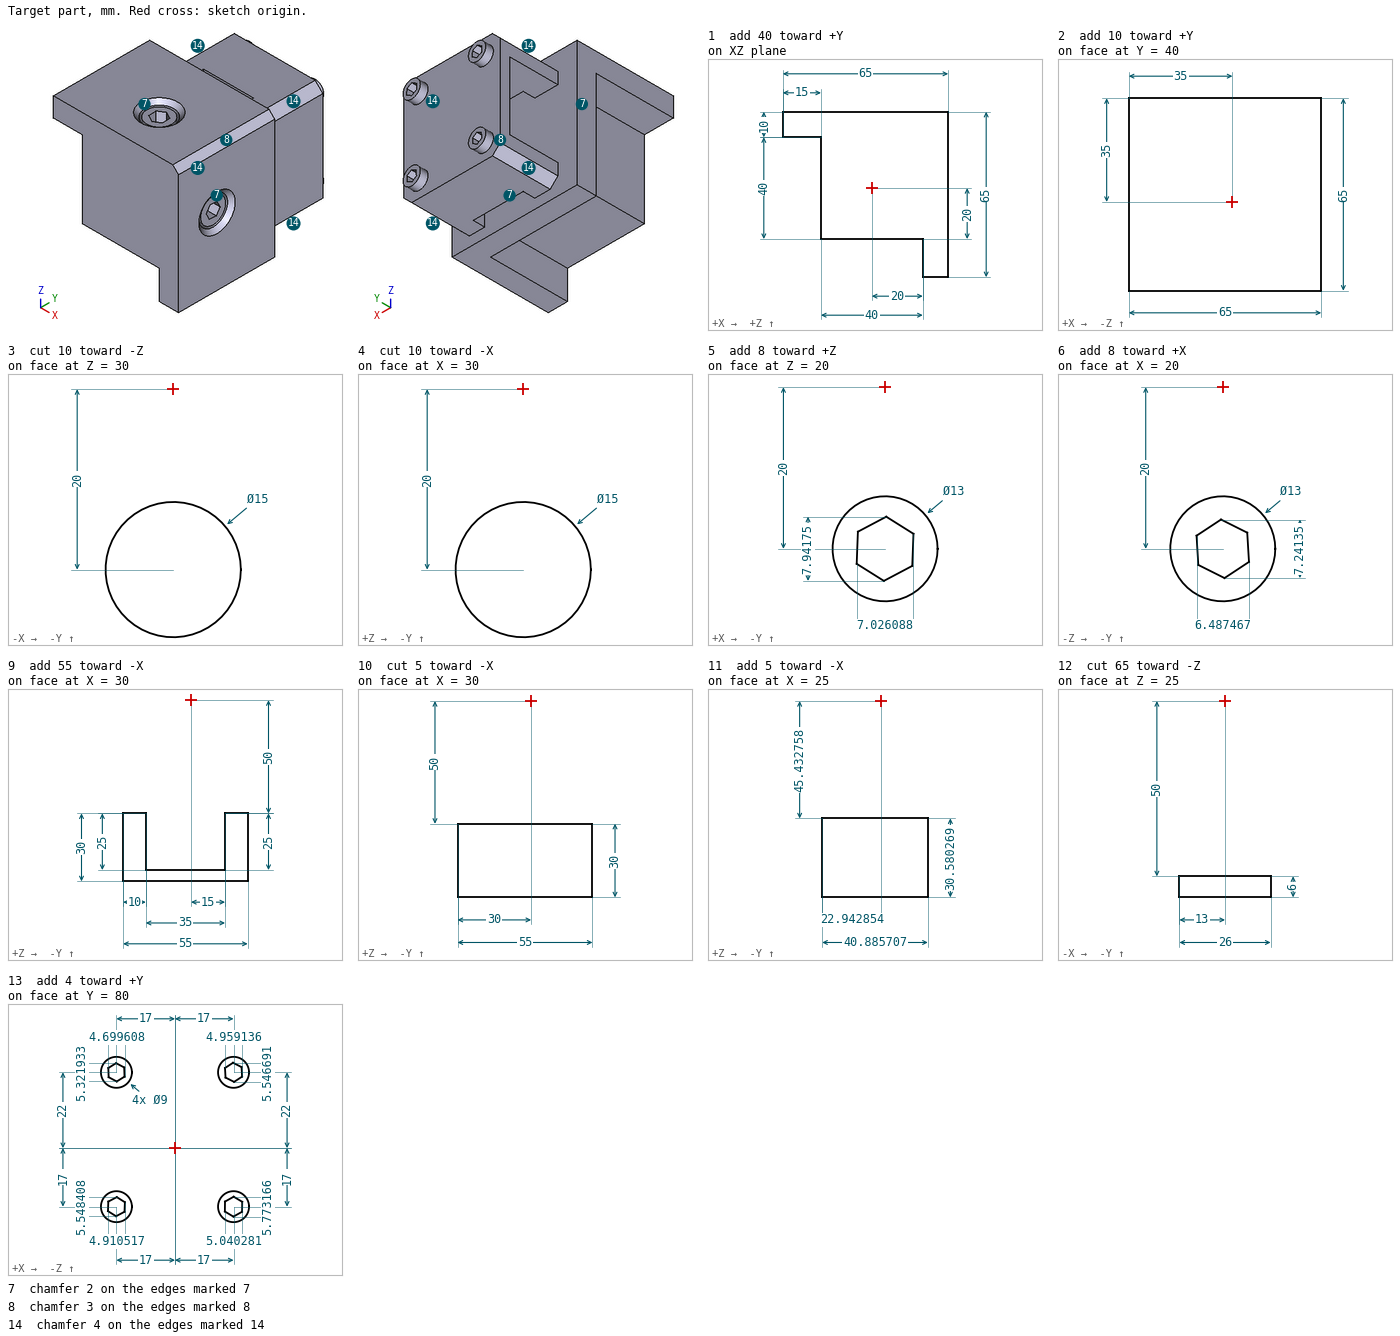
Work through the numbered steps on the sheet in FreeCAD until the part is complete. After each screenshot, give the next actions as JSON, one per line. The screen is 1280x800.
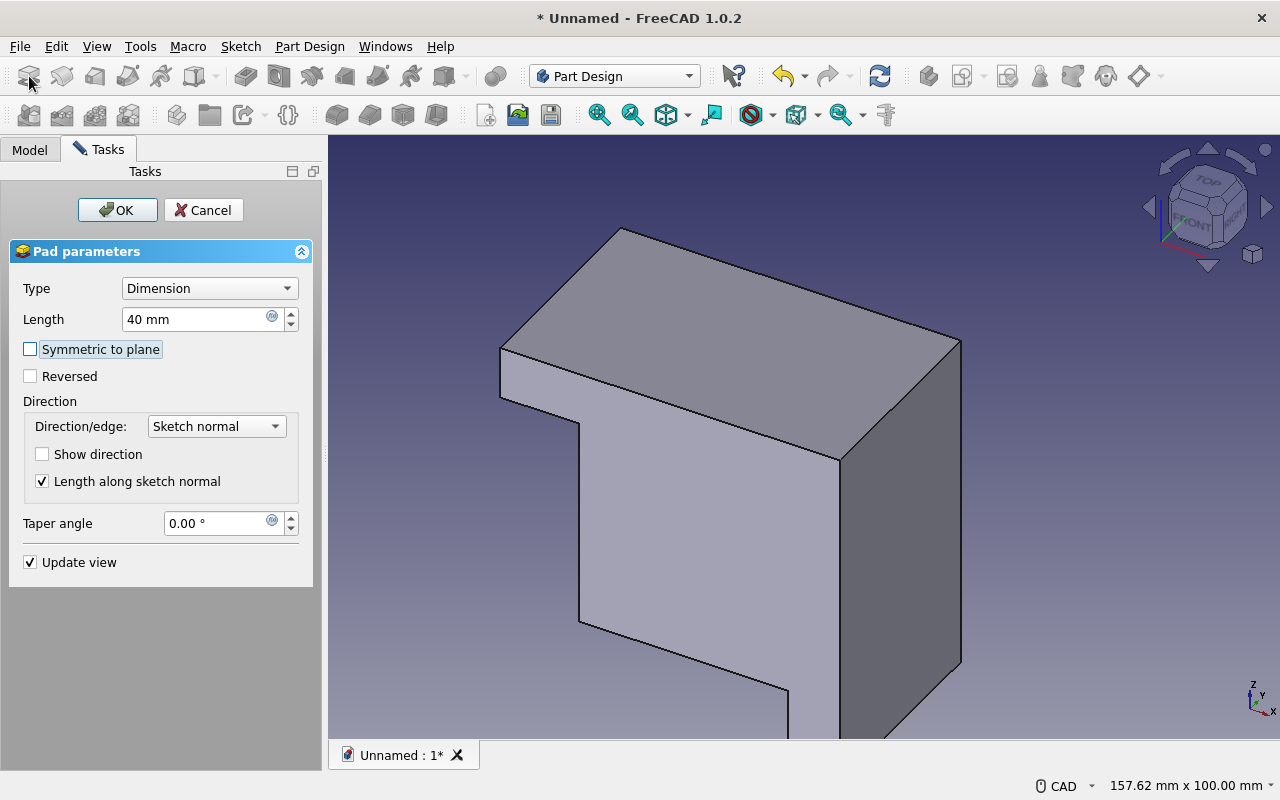
{"action": "left_click", "coordinate": [31, 376]}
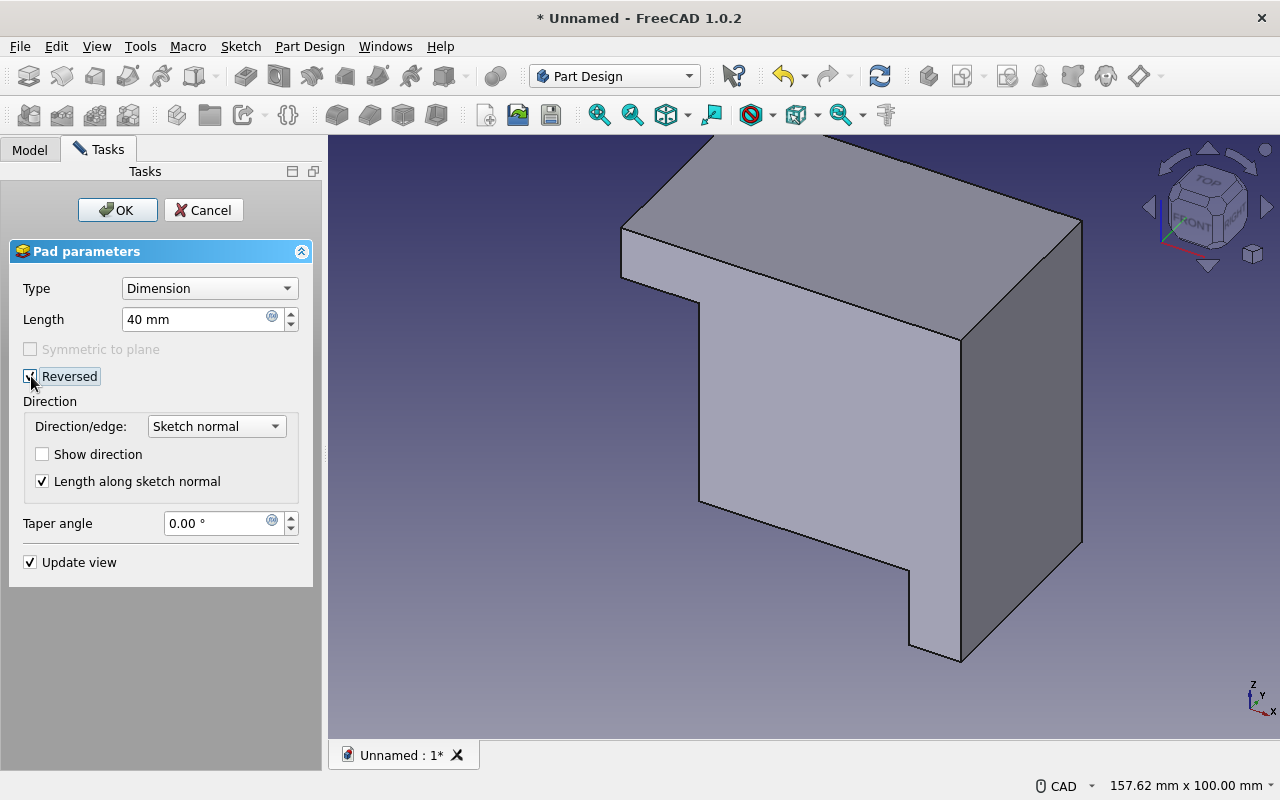
{"action": "left_click", "coordinate": [118, 210]}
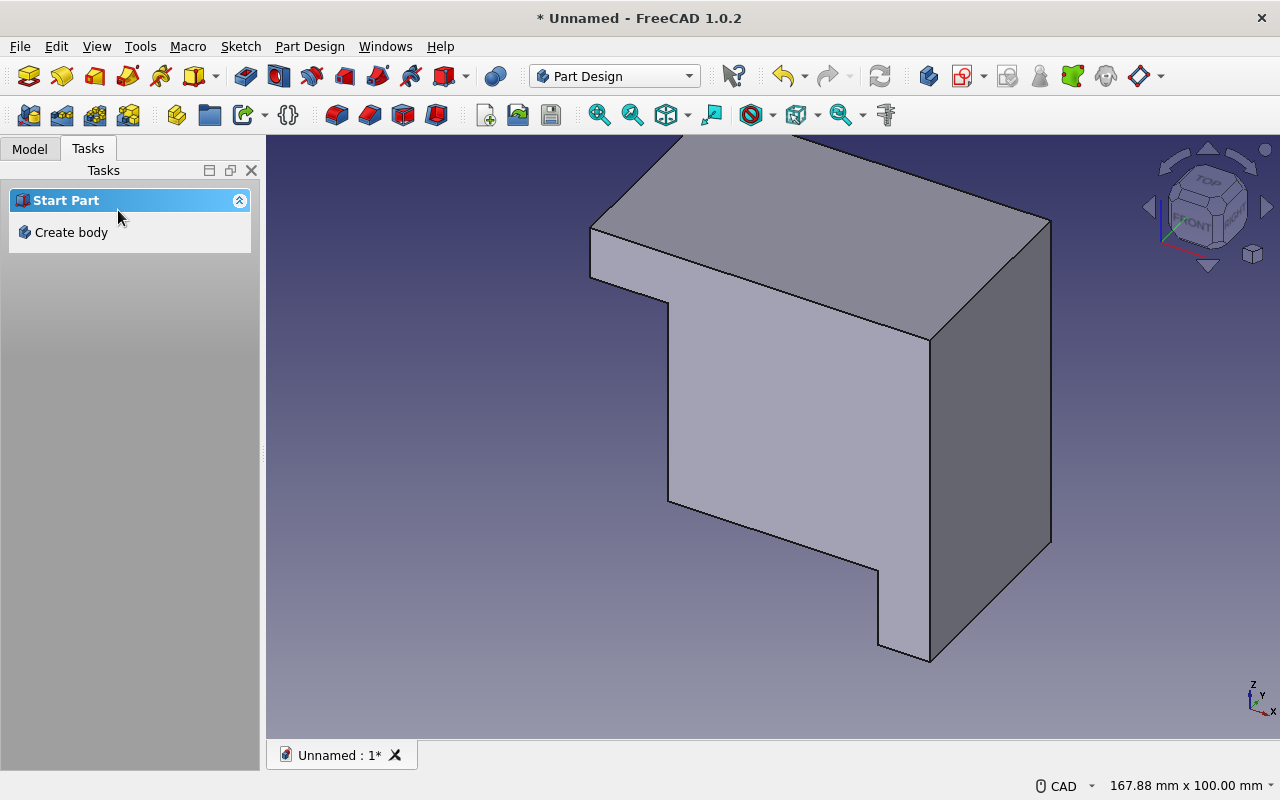
{"action": "left_click", "coordinate": [600, 116]}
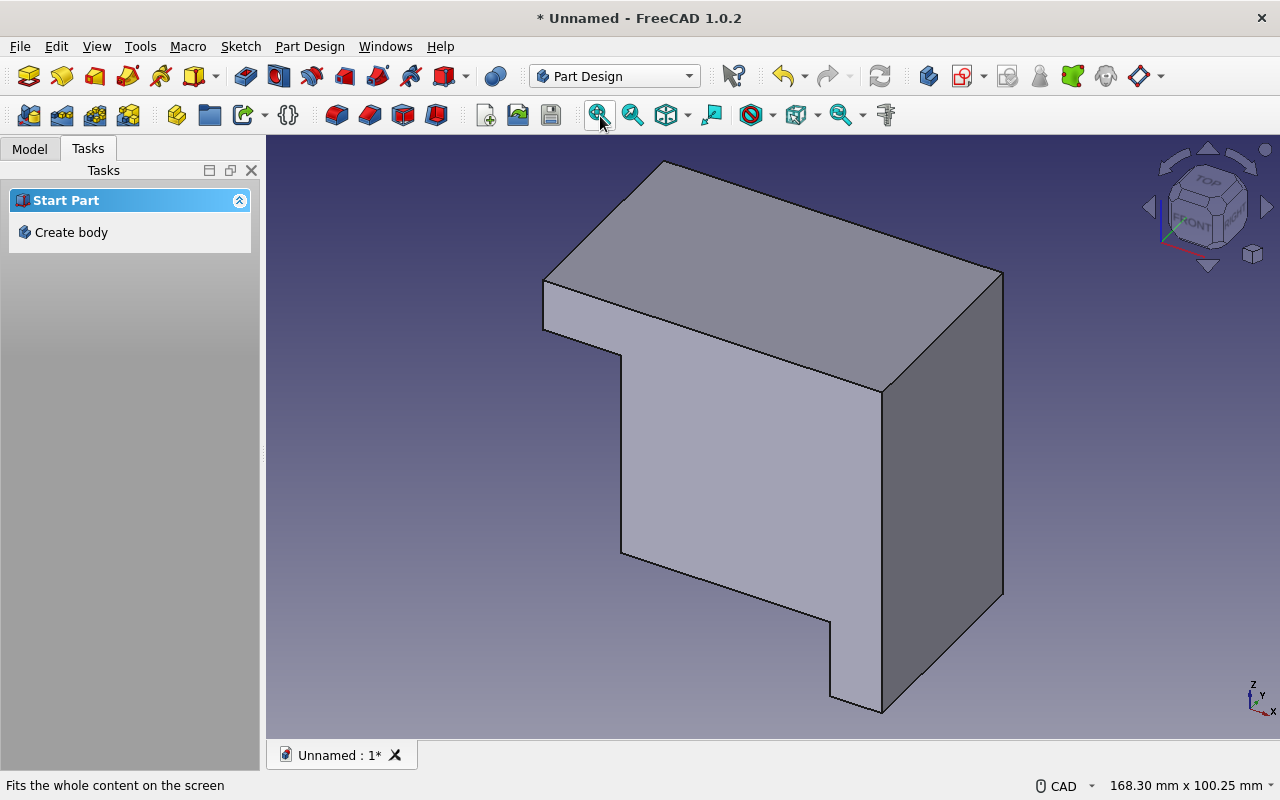
{"action": "key", "text": "4"}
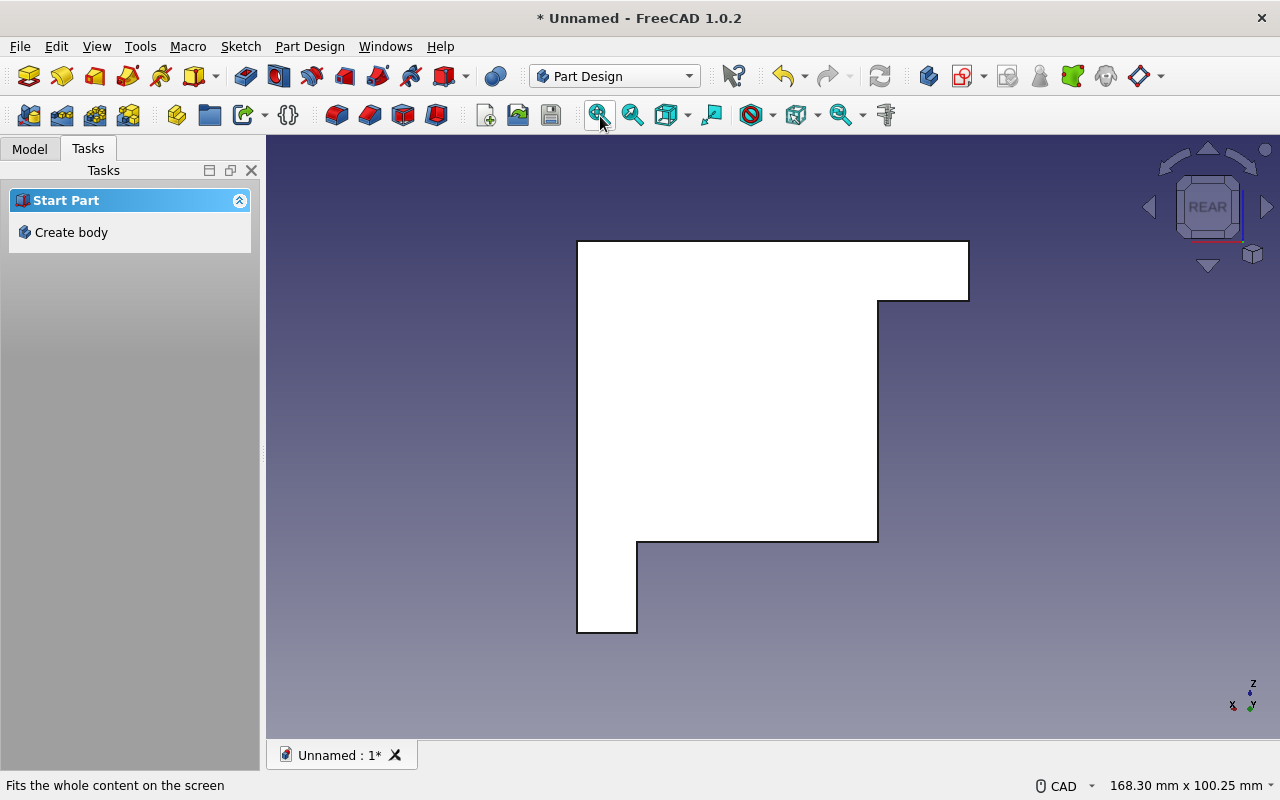
{"action": "left_click", "coordinate": [717, 380]}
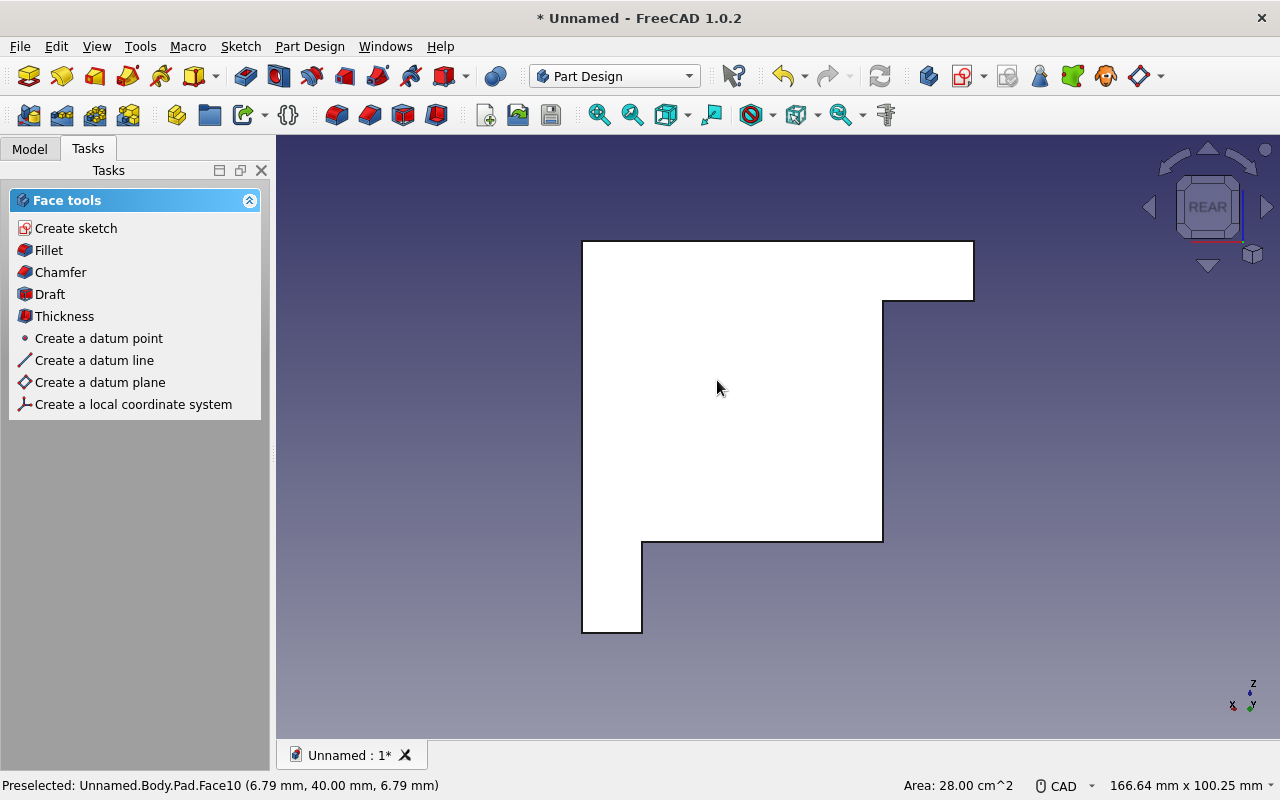
{"action": "left_click", "coordinate": [962, 76]}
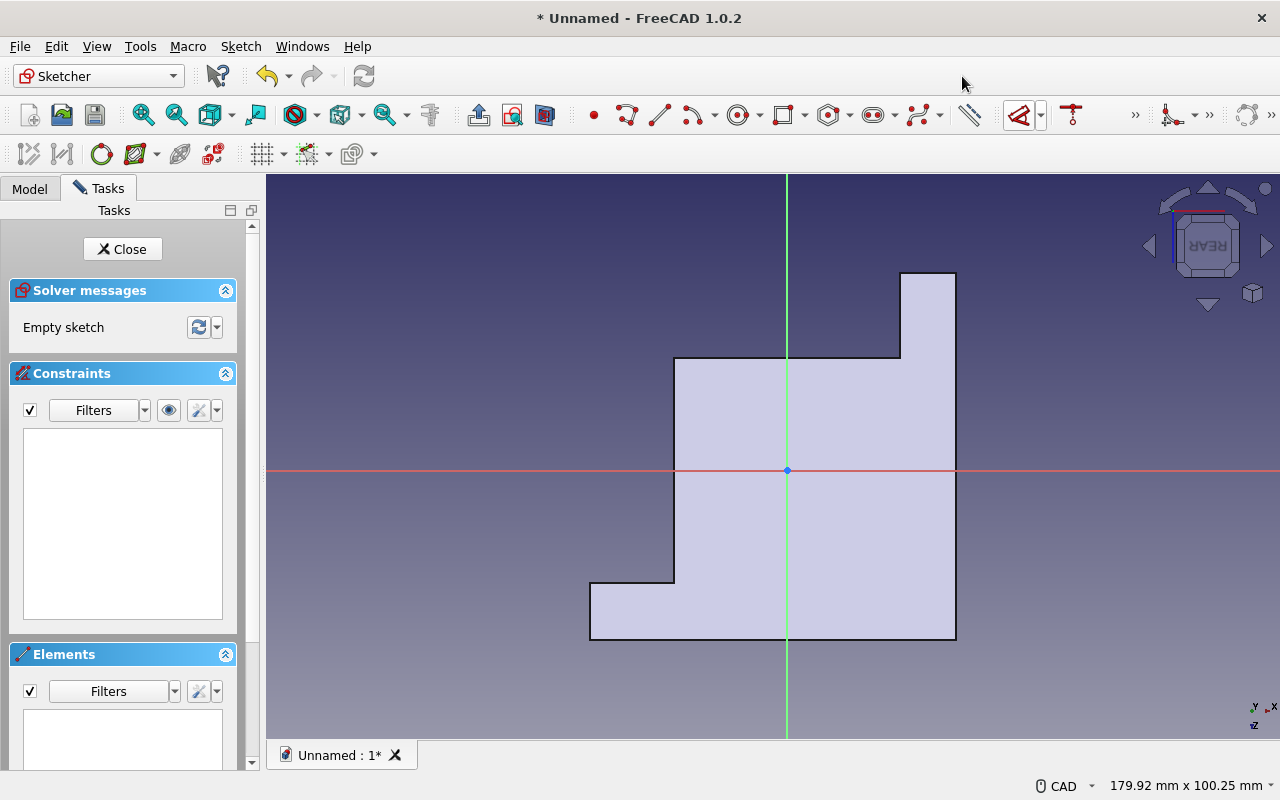
{"action": "left_click", "coordinate": [782, 116]}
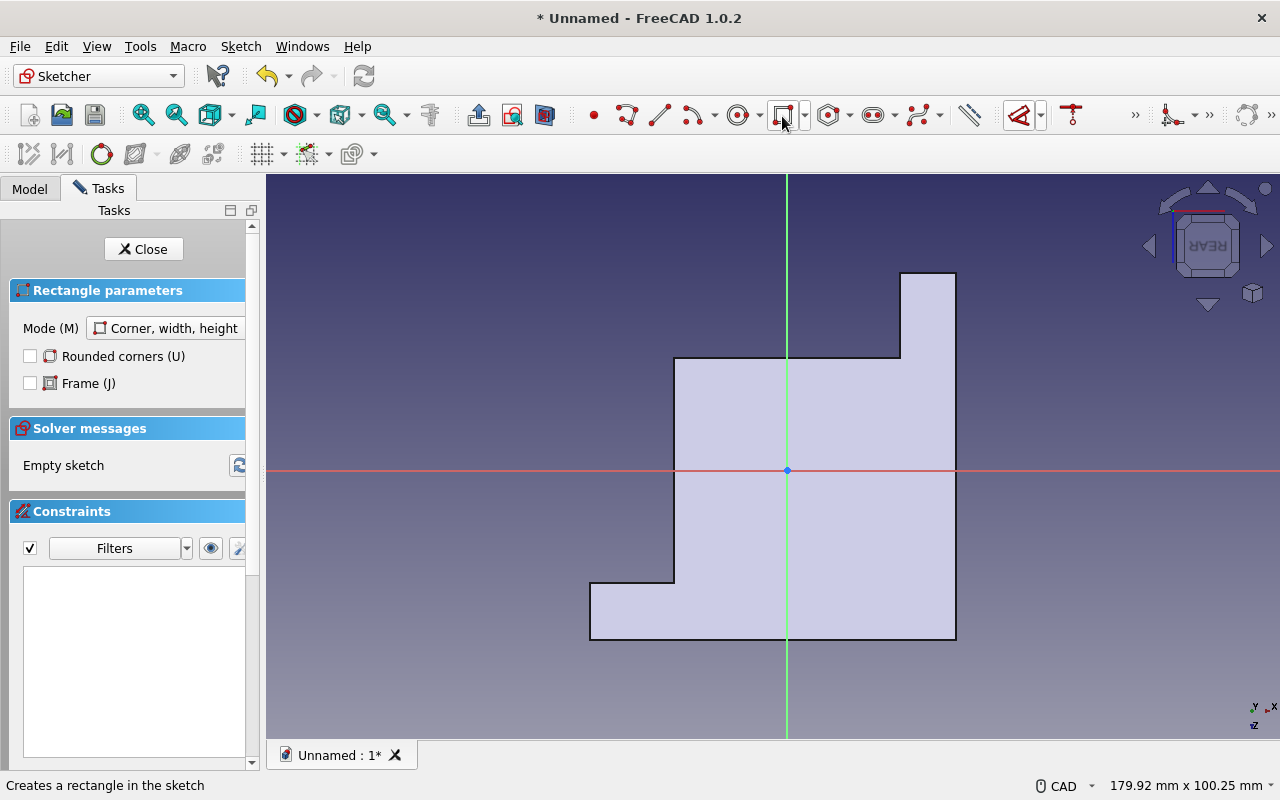
{"action": "left_click", "coordinate": [590, 273]}
{"action": "mouse_move", "coordinate": [956, 640]}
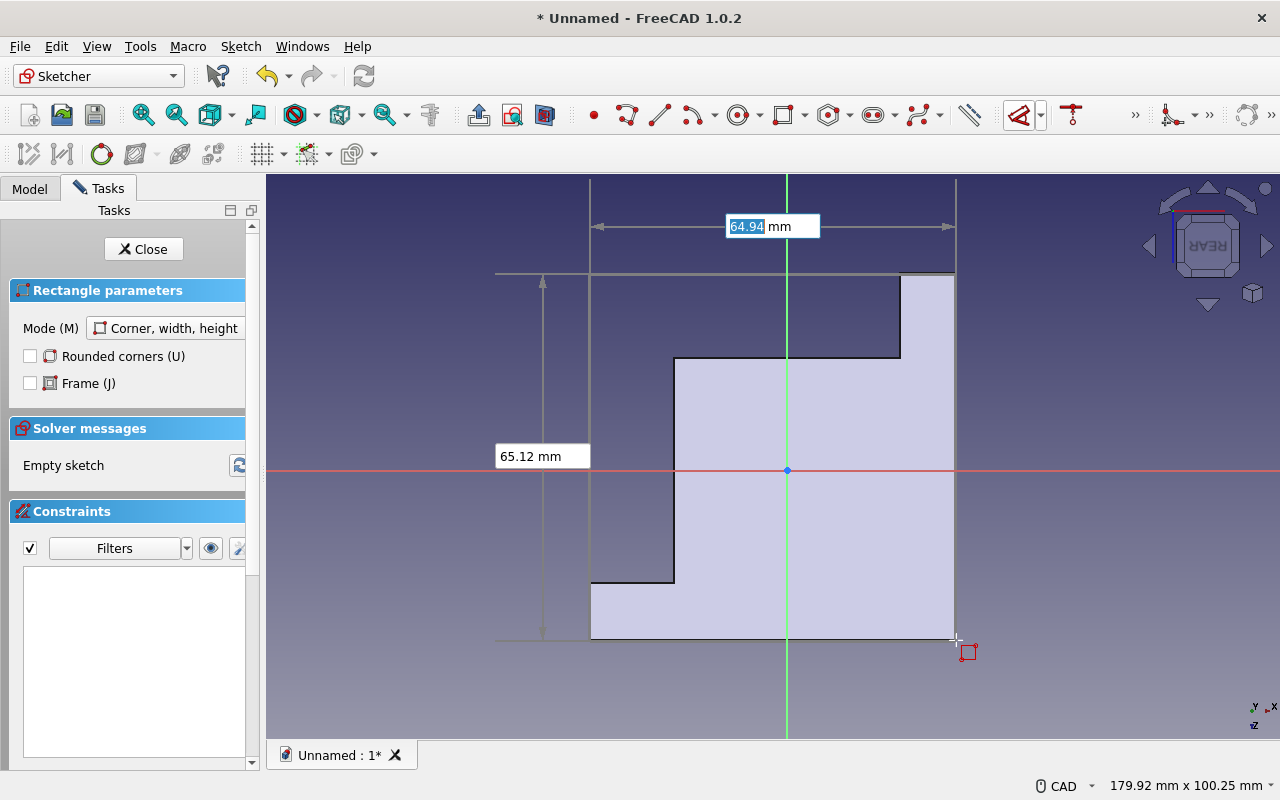
{"action": "type", "text": "65"}
{"action": "key", "text": "Tab"}
{"action": "type", "text": "65"}
{"action": "key", "text": "Return"}
{"action": "key", "text": "Escape"}